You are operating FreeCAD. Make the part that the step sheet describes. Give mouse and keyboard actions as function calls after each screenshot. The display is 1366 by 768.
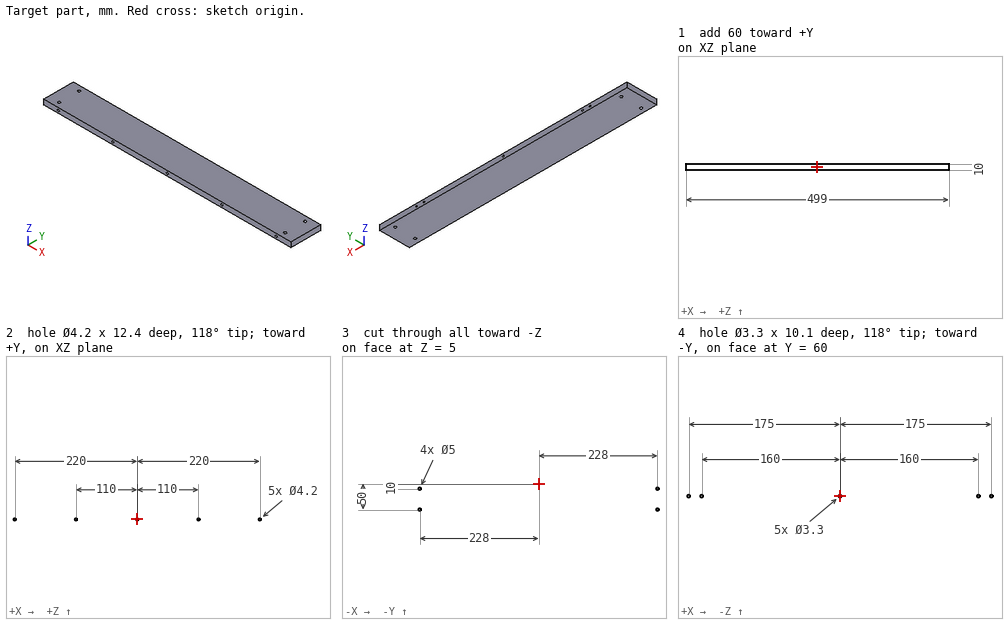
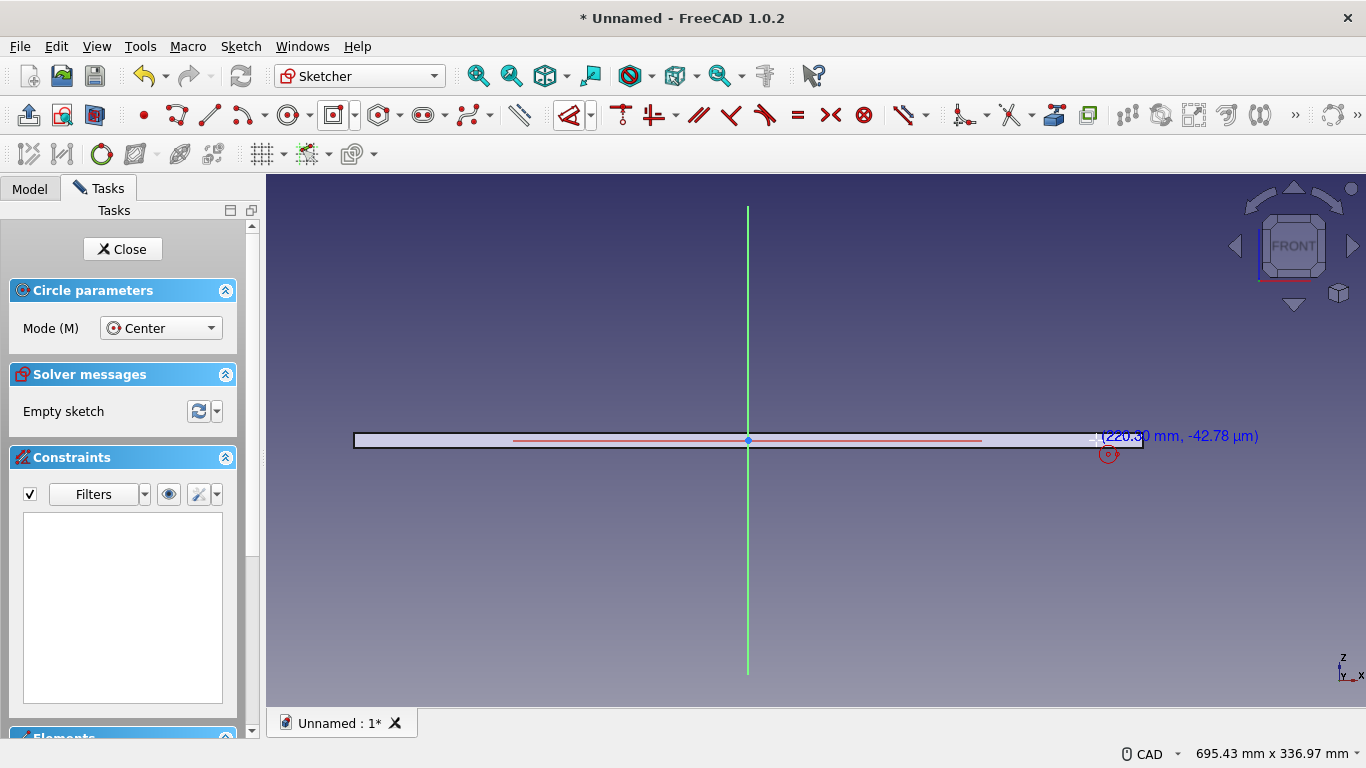
click(1096, 440)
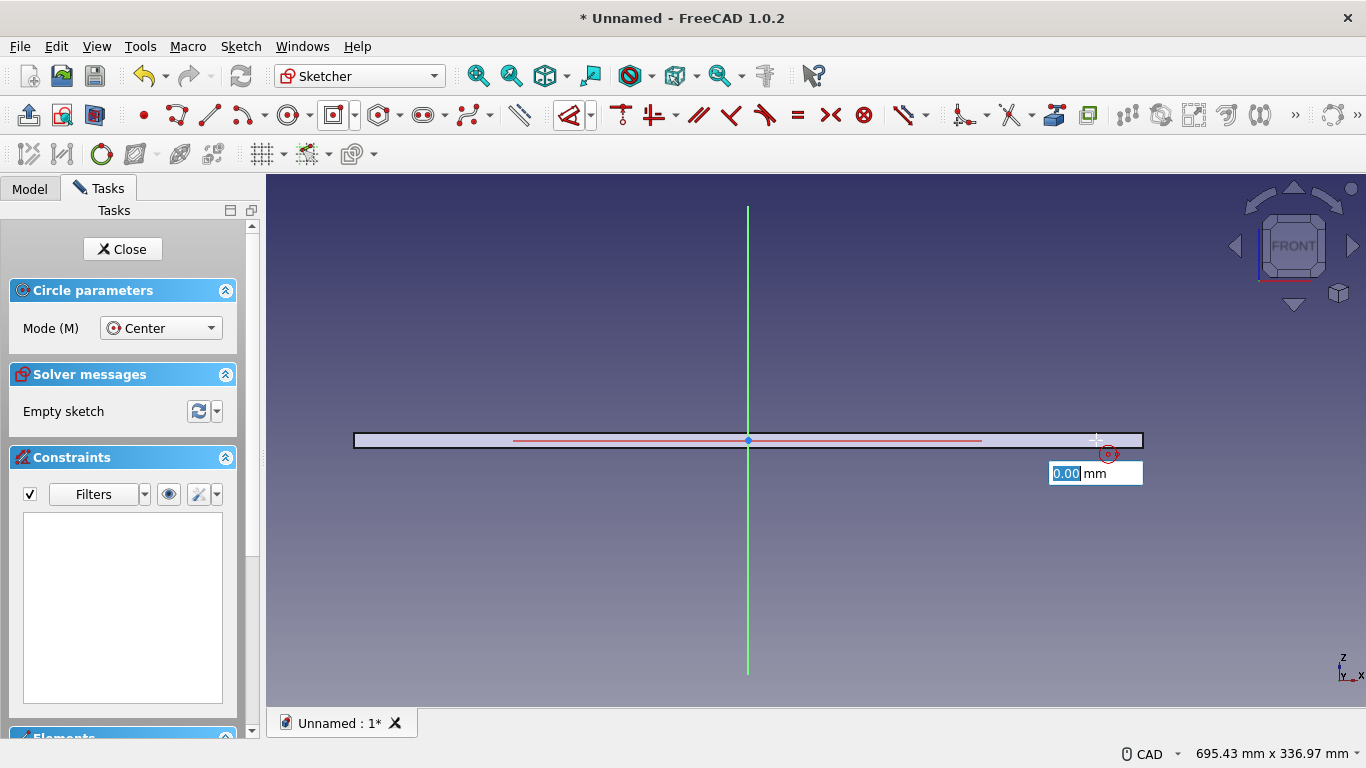
scroll(1095, 444, up, 9)
move(1091, 439)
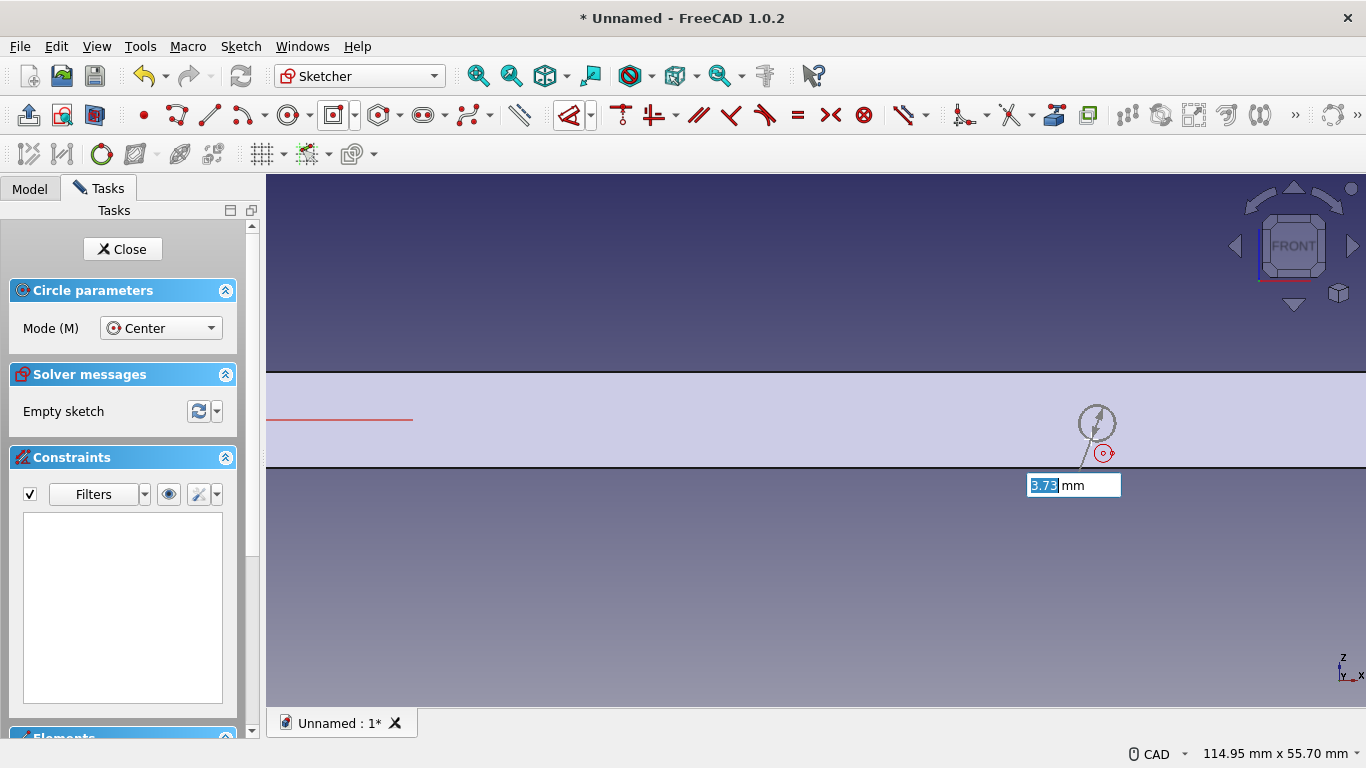
text(4.2)
key(Return)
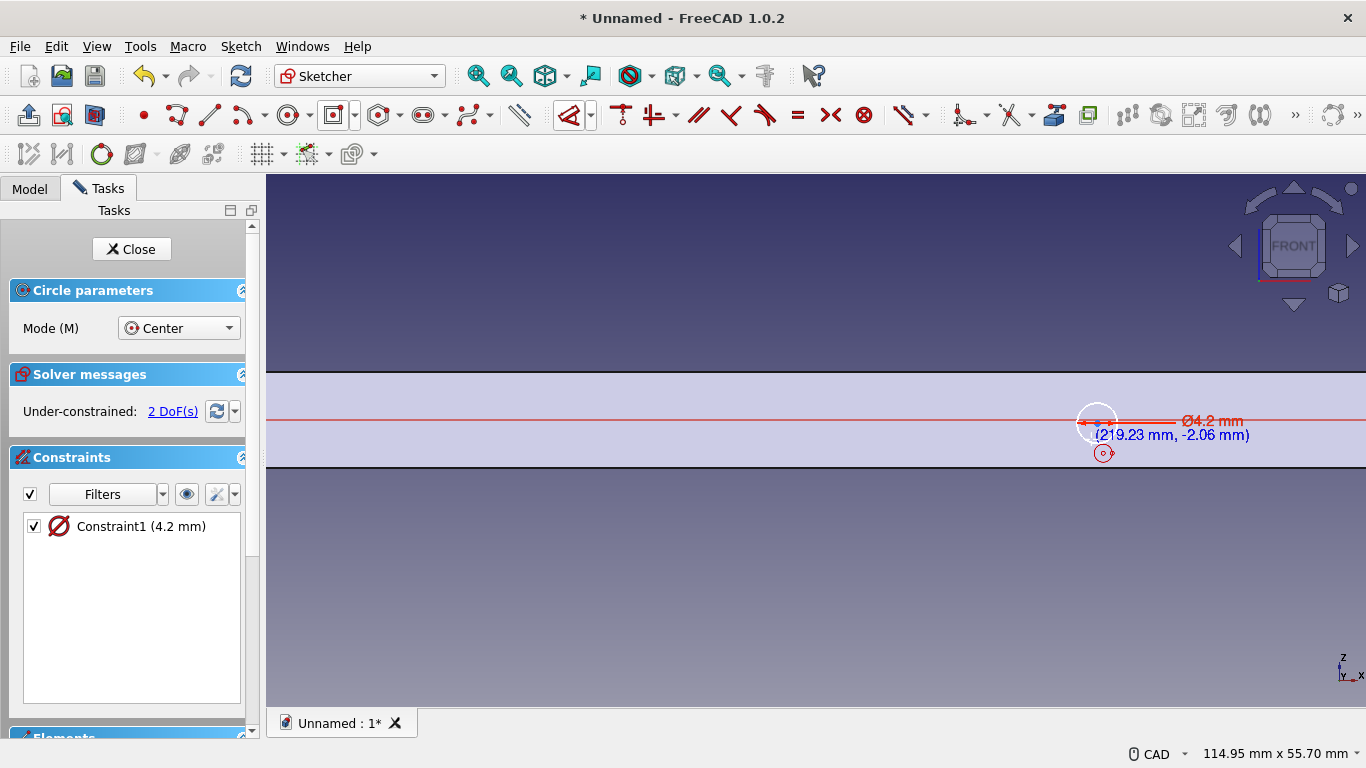
scroll(1095, 445, down, 9)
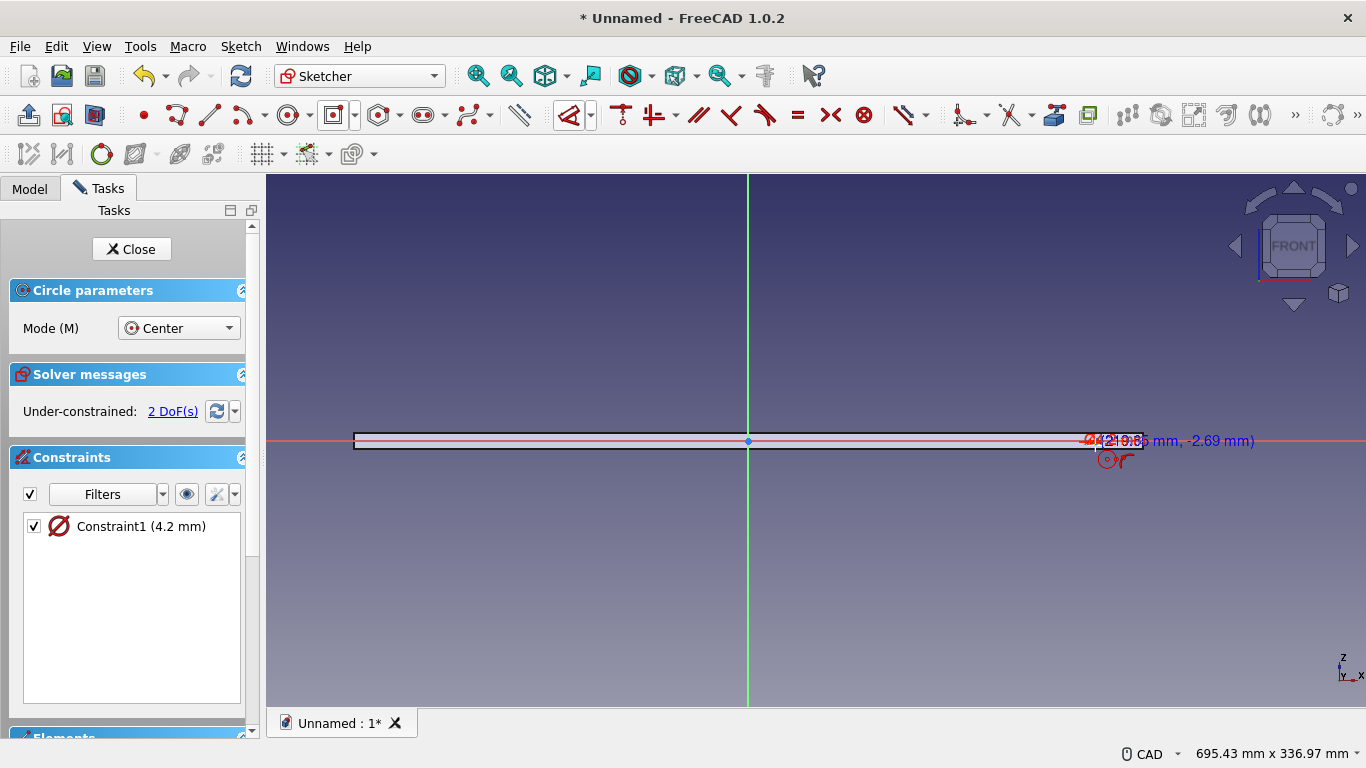
scroll(922, 441, up, 10)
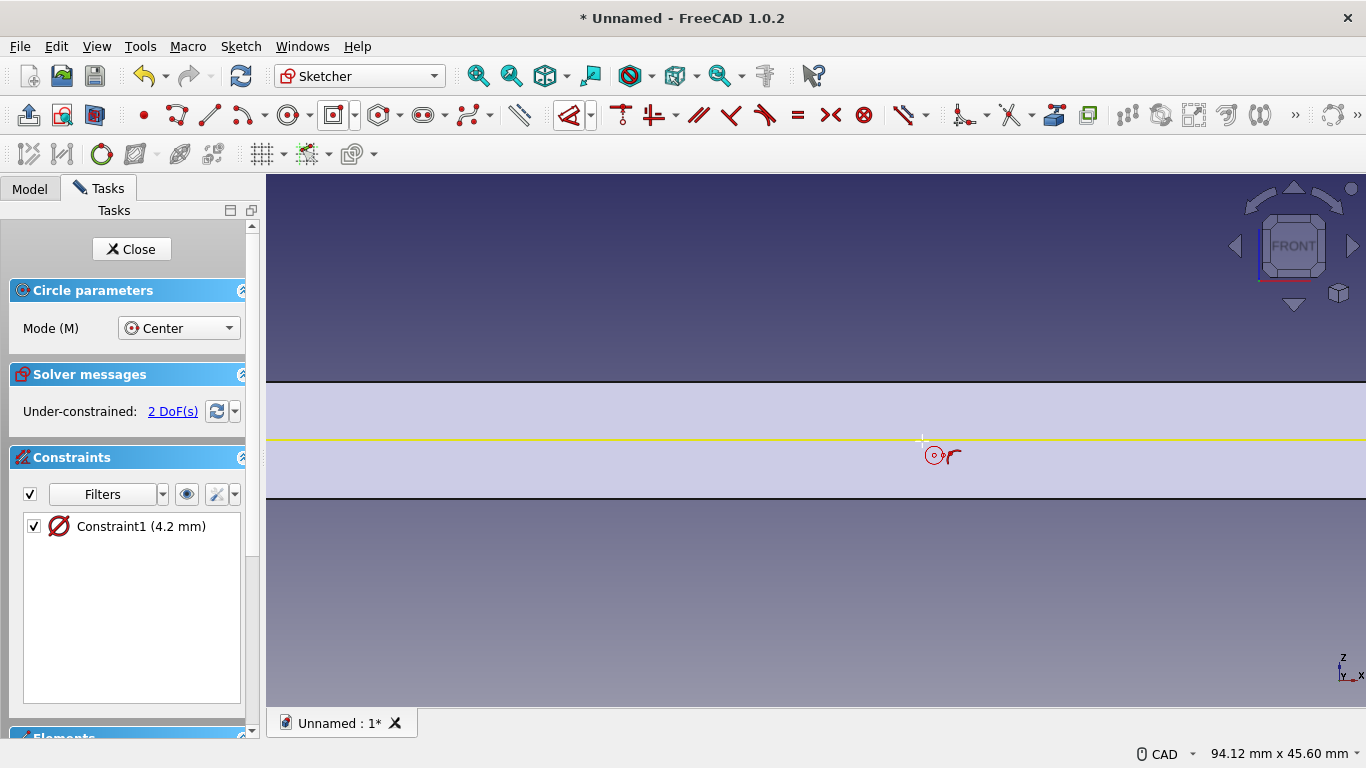
scroll(922, 441, down, 10)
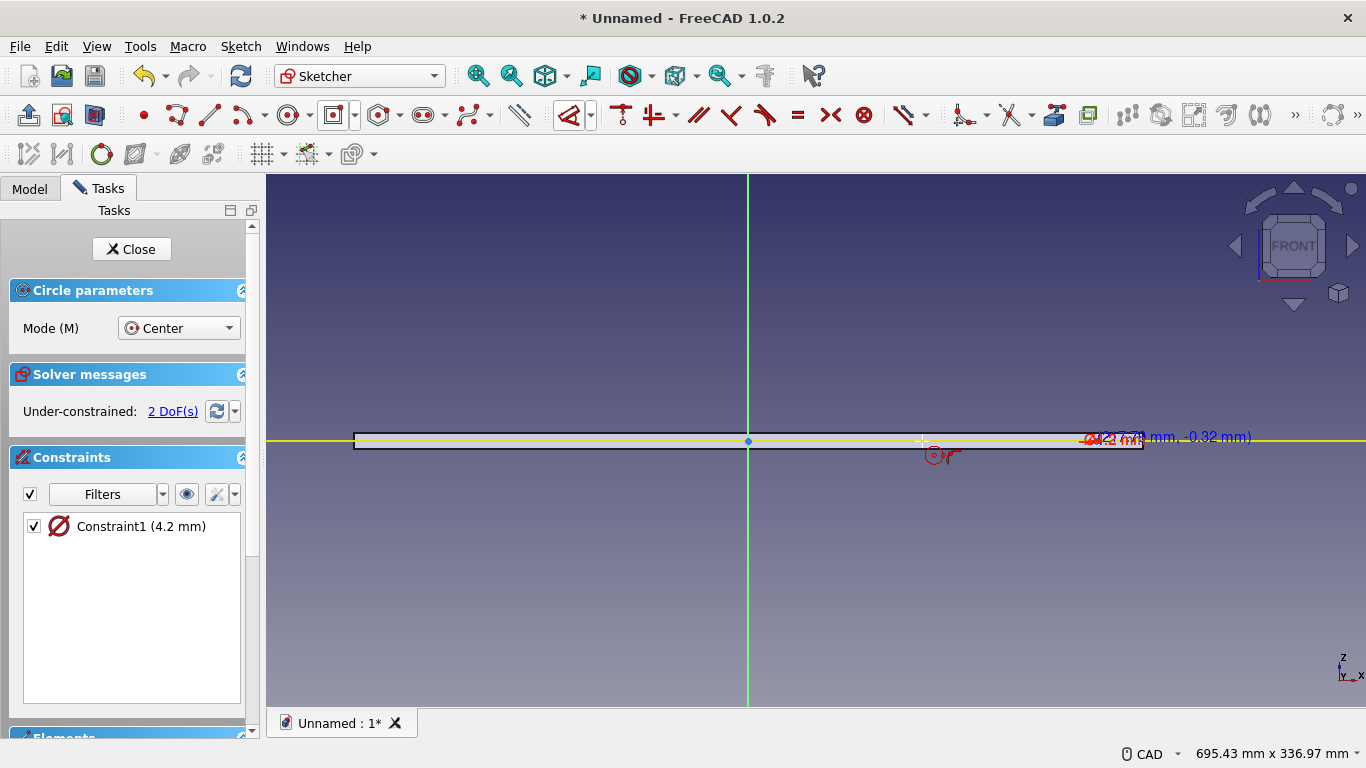
click(922, 441)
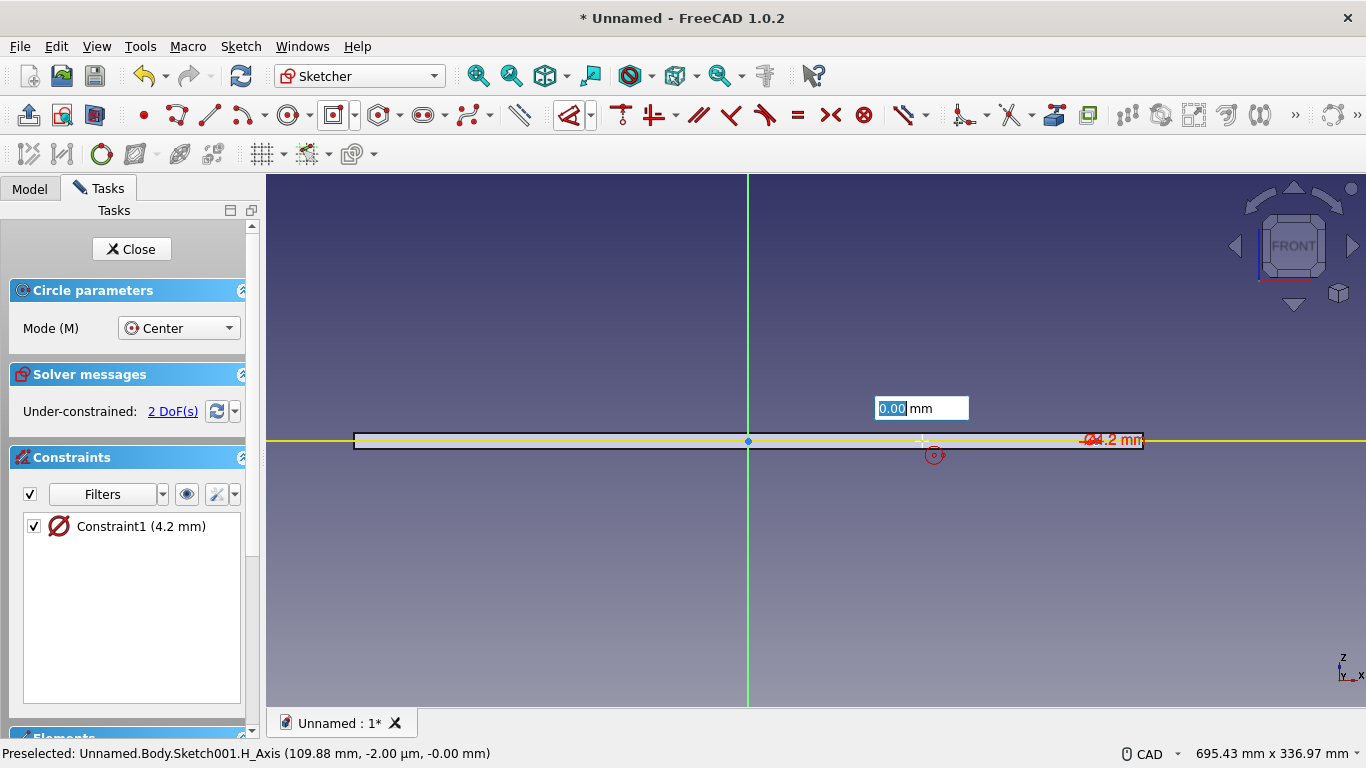
scroll(921, 444, up, 9)
move(918, 444)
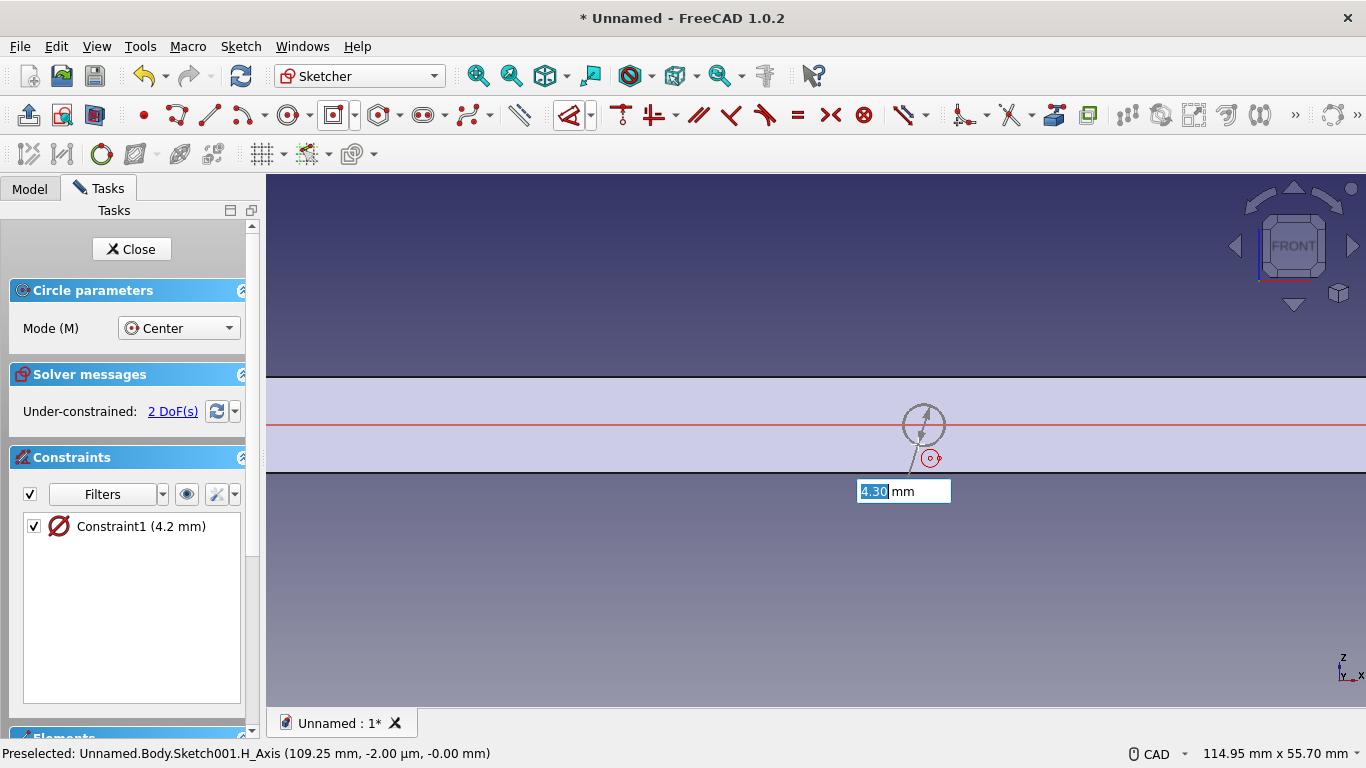
text(4.2)
key(Return)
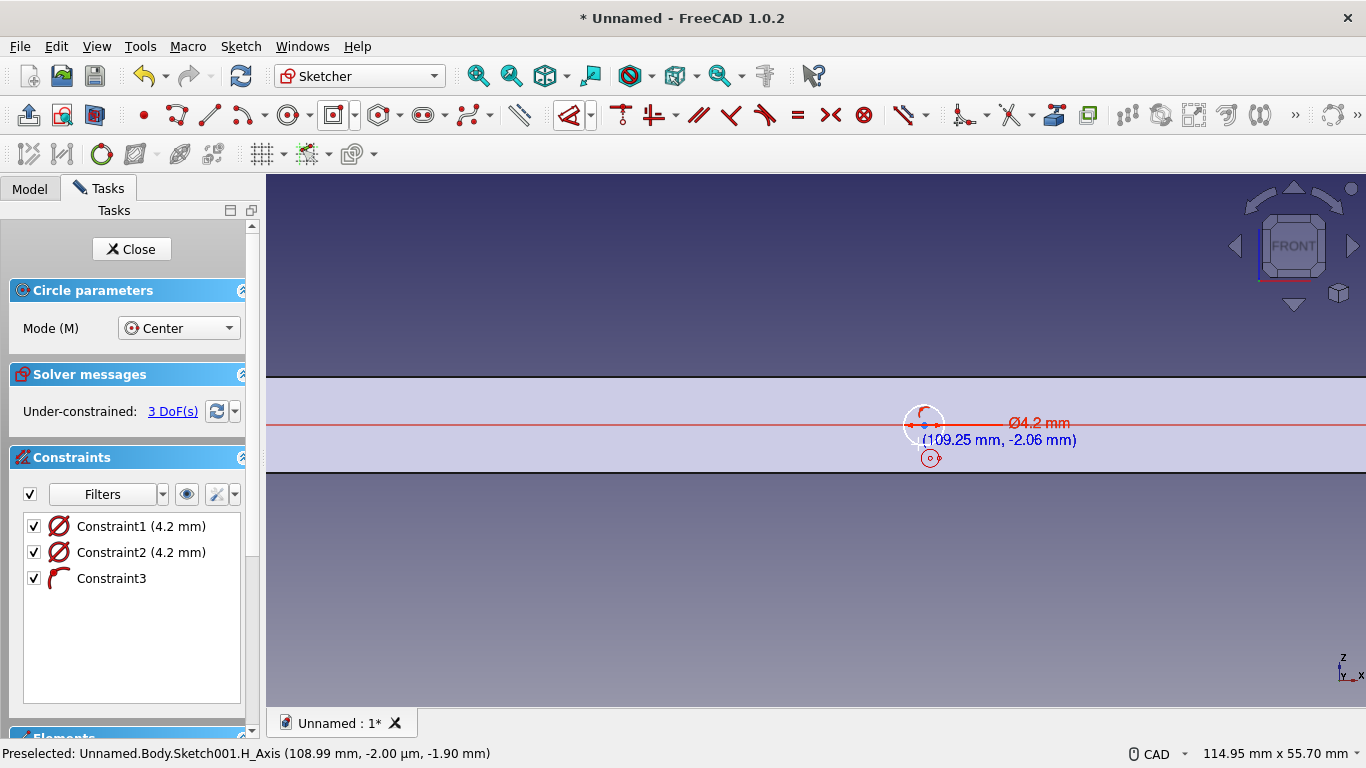
scroll(921, 444, down, 9)